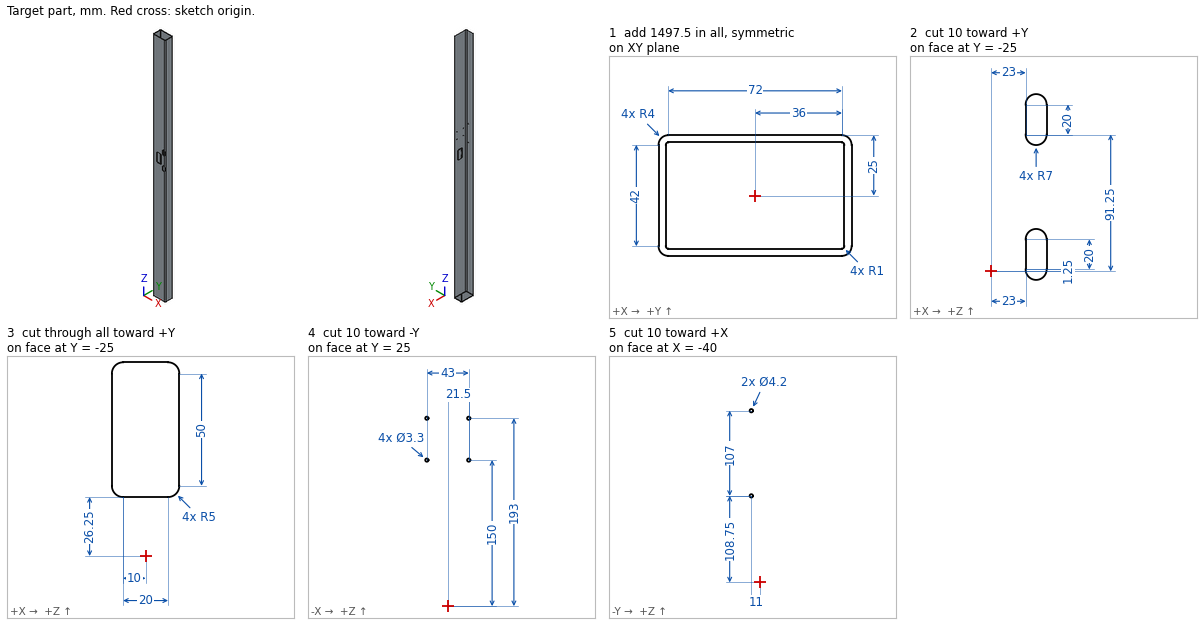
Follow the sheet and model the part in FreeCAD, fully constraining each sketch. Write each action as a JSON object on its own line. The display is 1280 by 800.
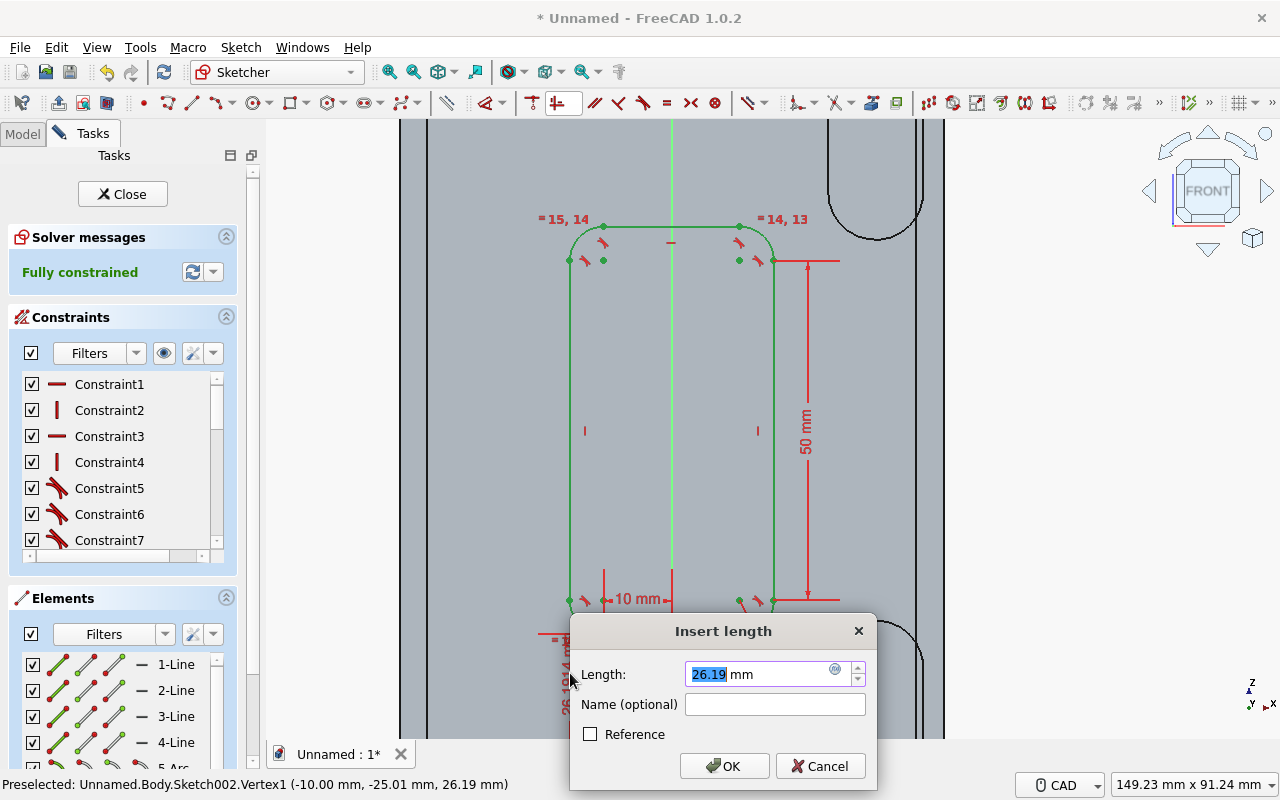
{"action": "type", "text": "26.25"}
{"action": "key", "text": "Return"}
{"action": "key", "text": "Escape"}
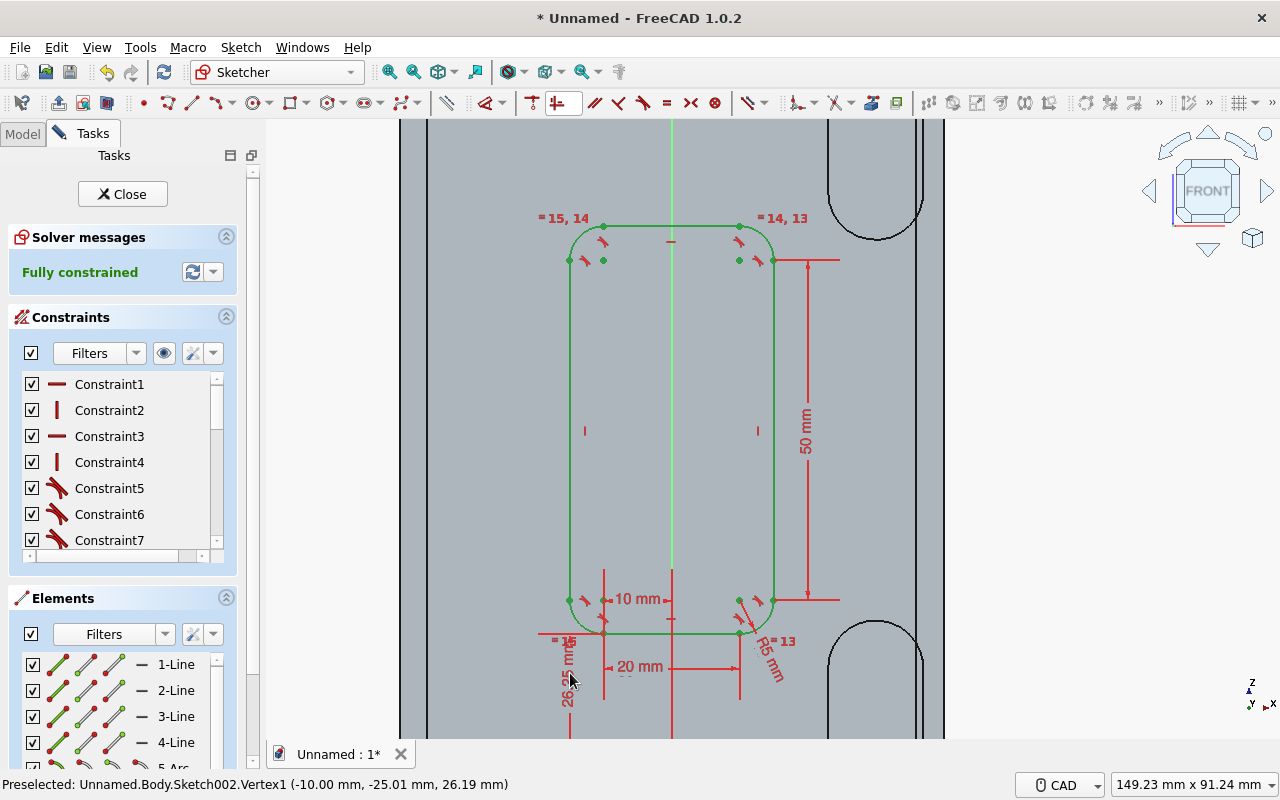
{"action": "left_click", "coordinate": [123, 194]}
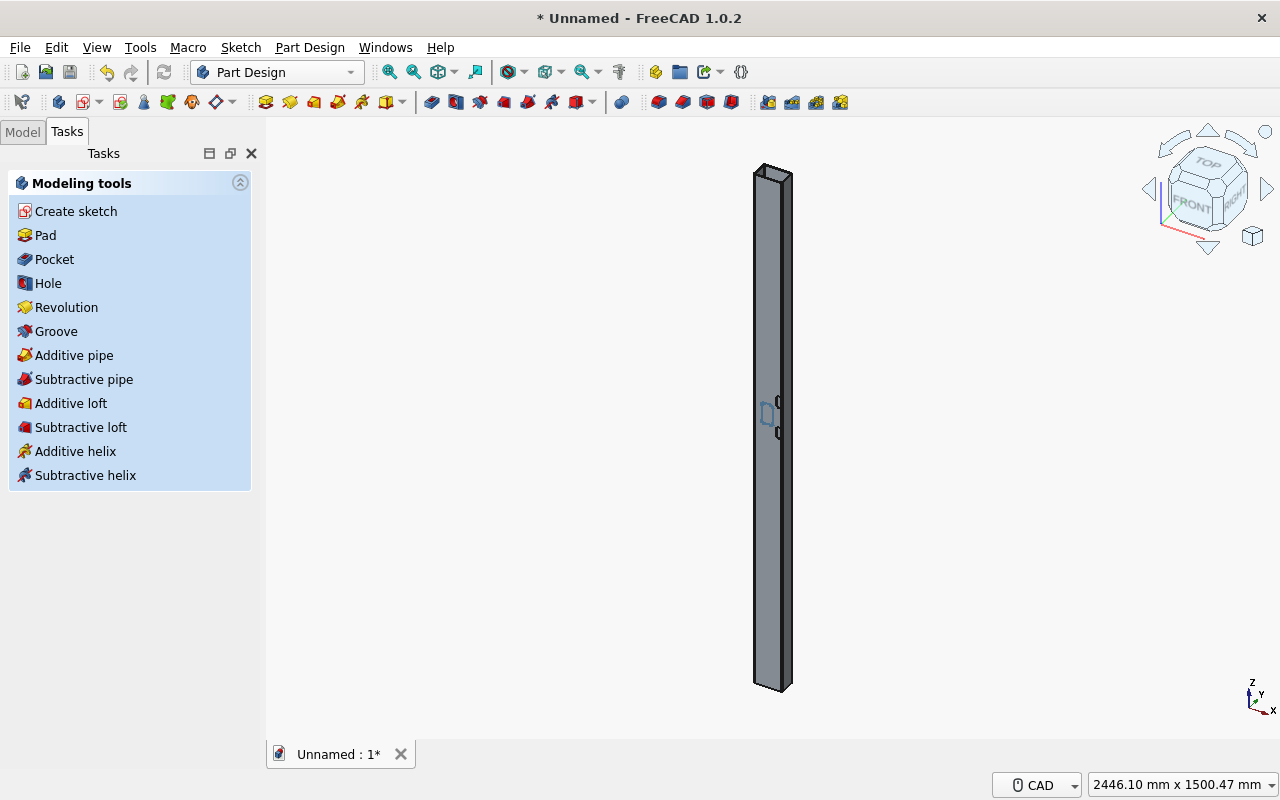
{"action": "left_click", "coordinate": [432, 102]}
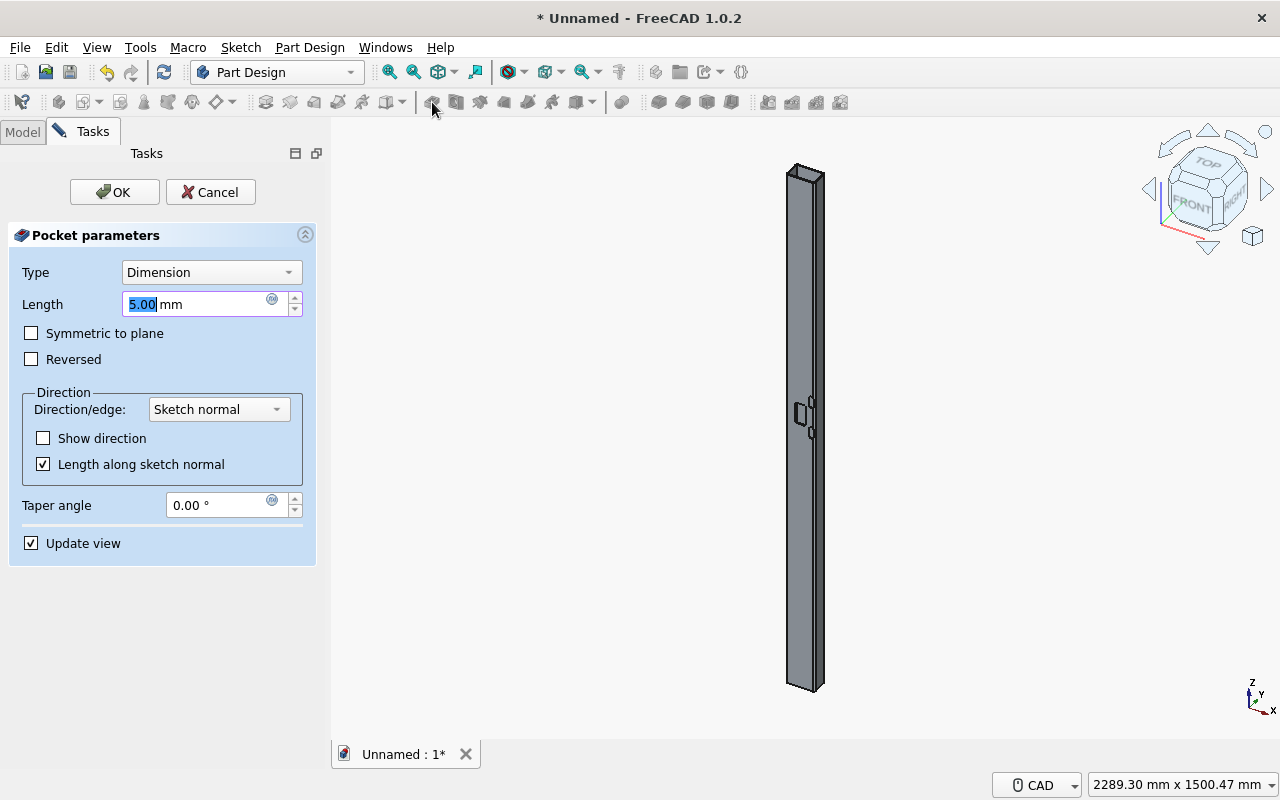
{"action": "left_click", "coordinate": [212, 272]}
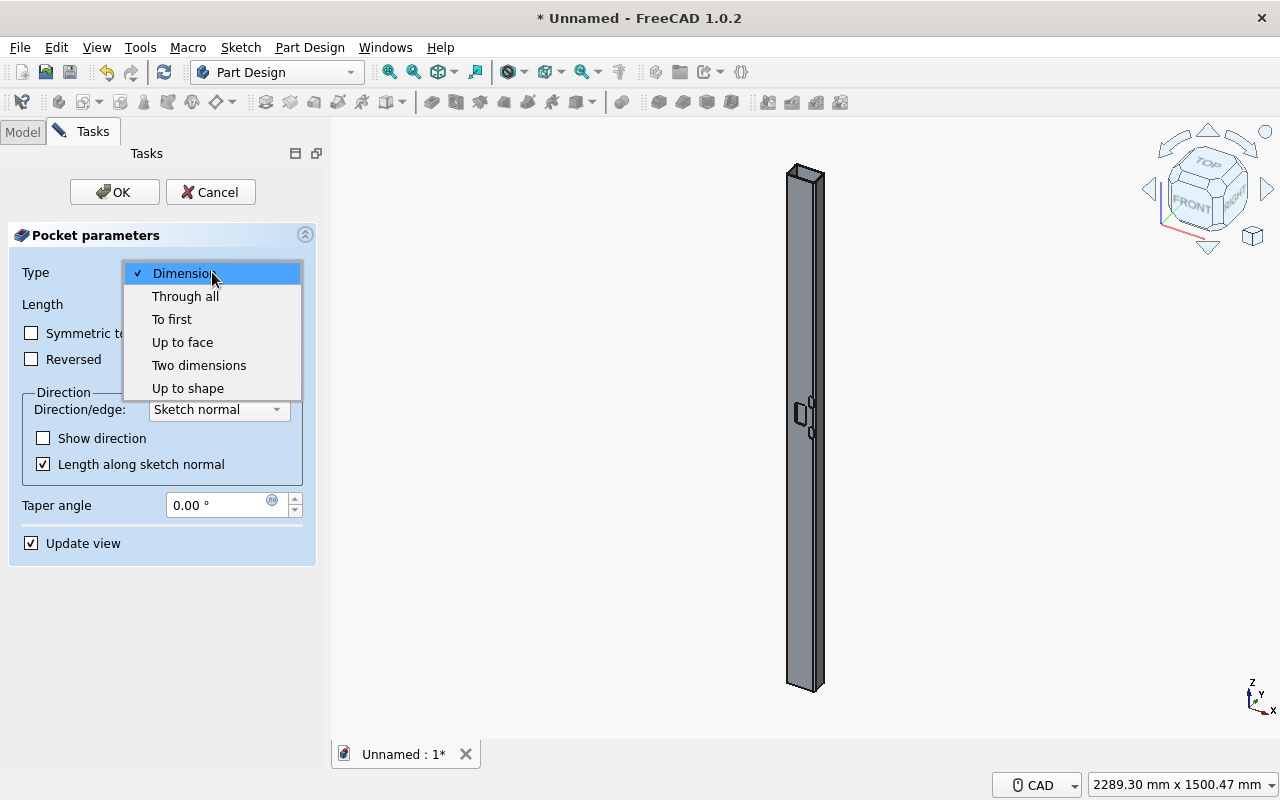
{"action": "left_click", "coordinate": [212, 296]}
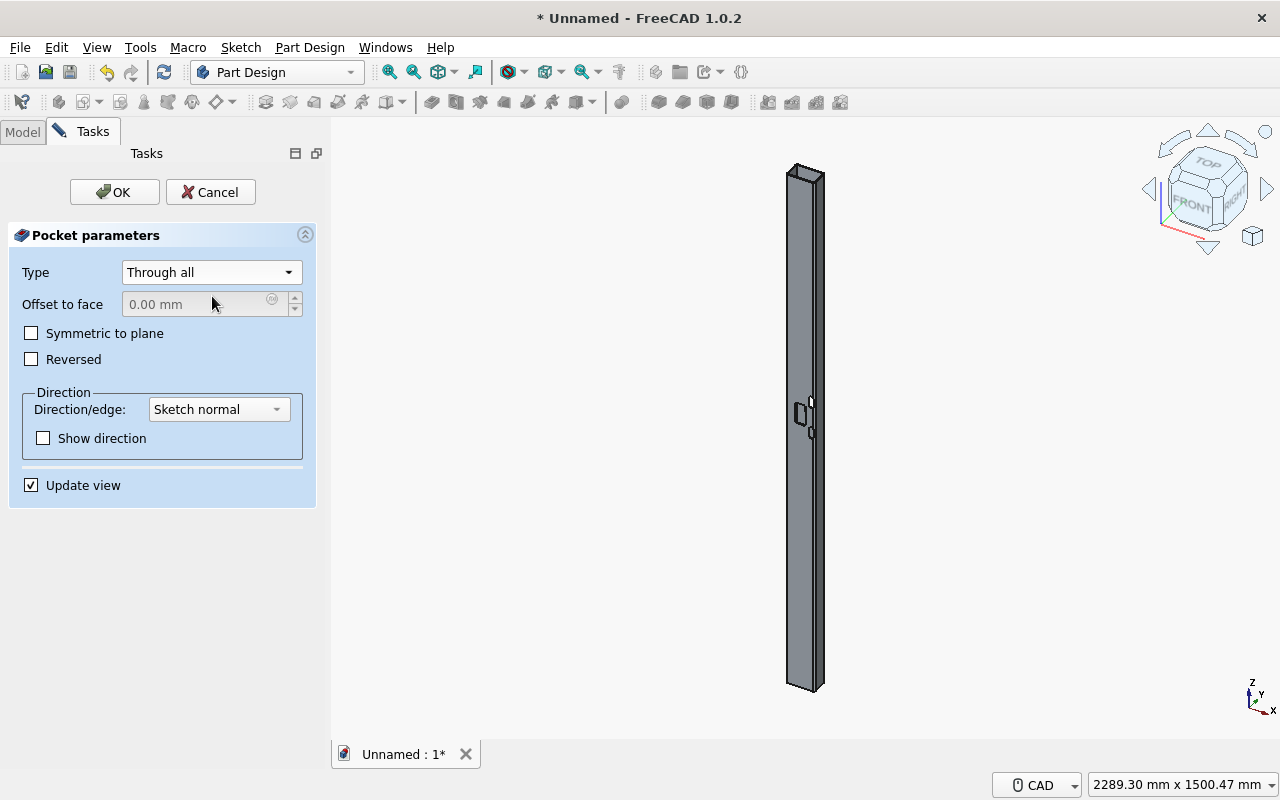
{"action": "left_click", "coordinate": [115, 192]}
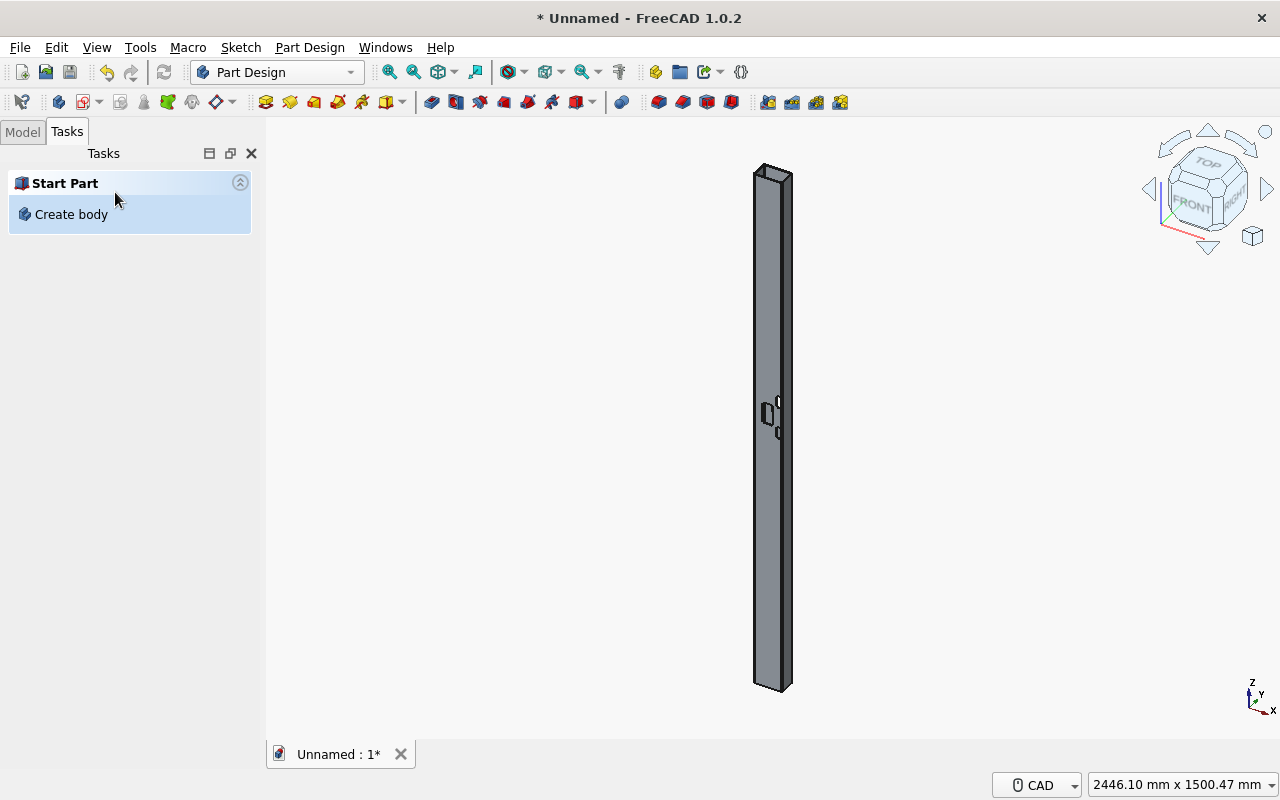
{"action": "key", "text": "4"}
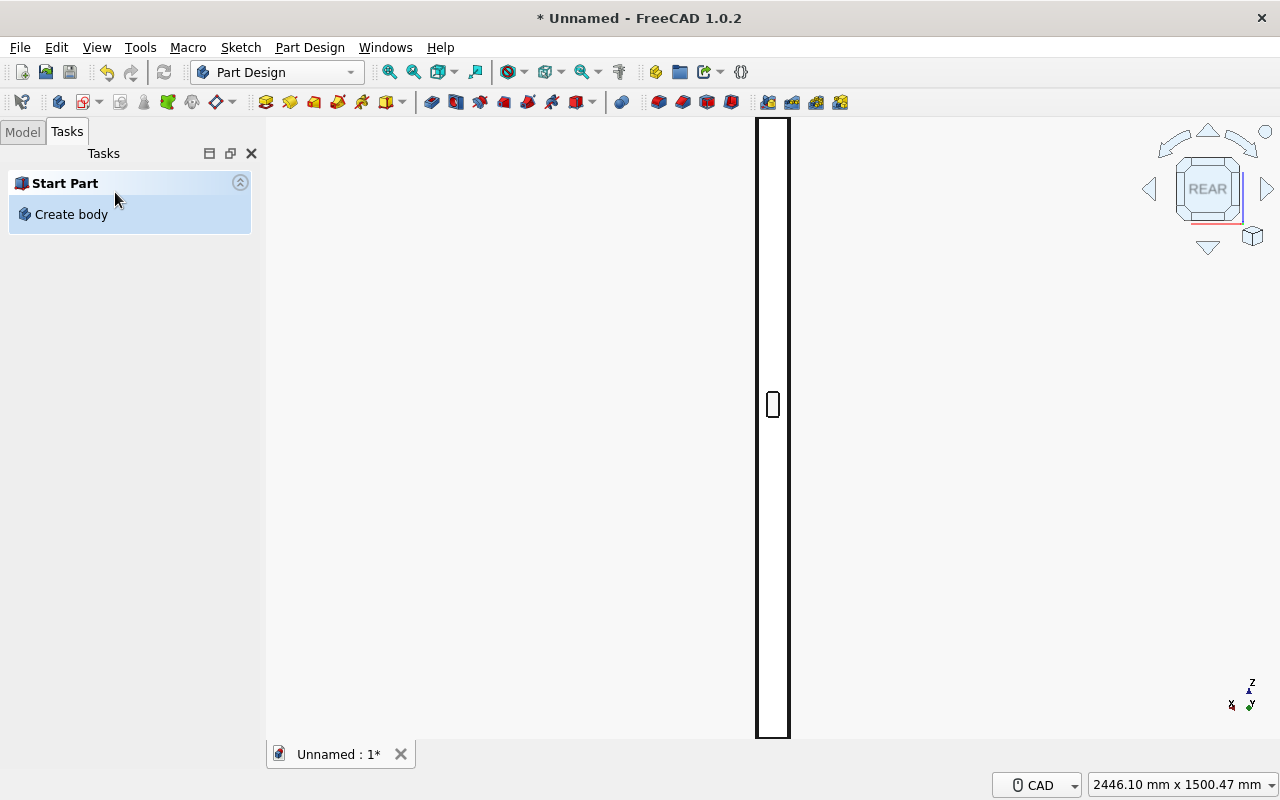
{"action": "left_click", "coordinate": [773, 161]}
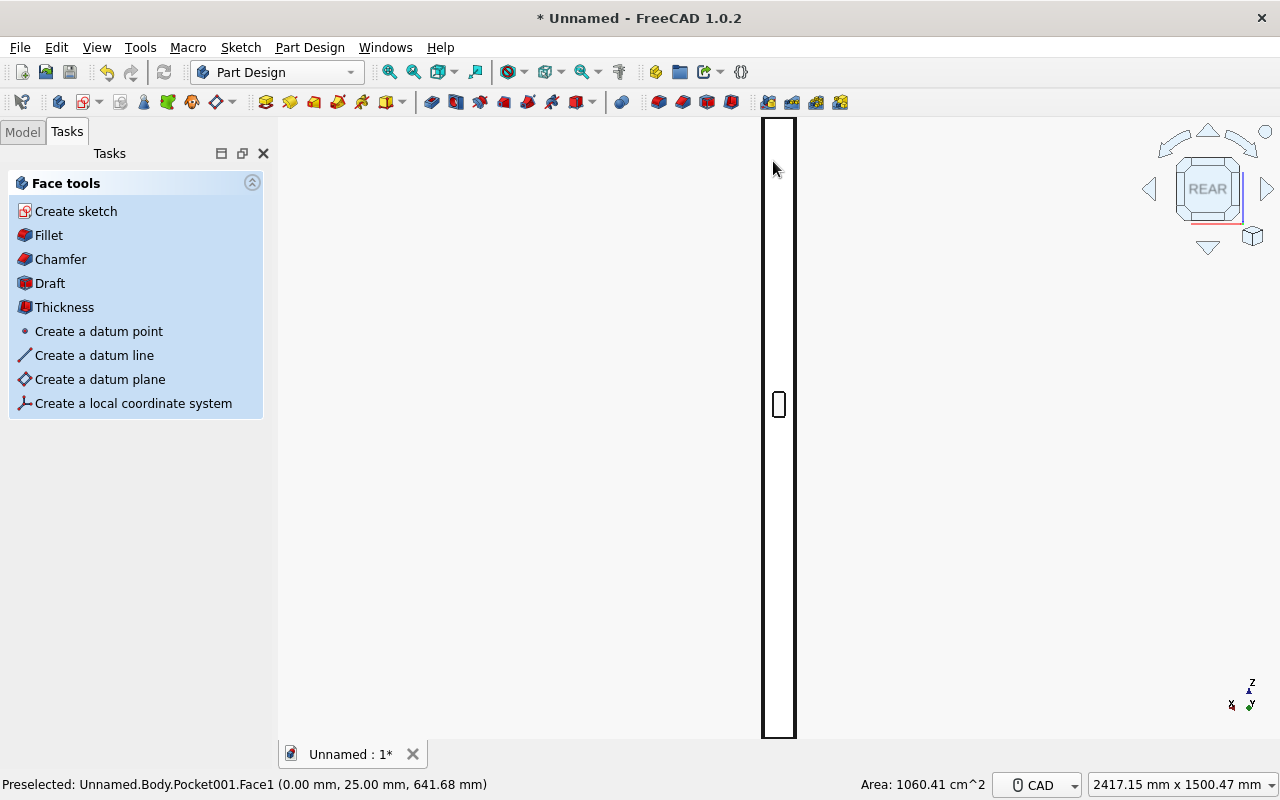
{"action": "left_click", "coordinate": [84, 102]}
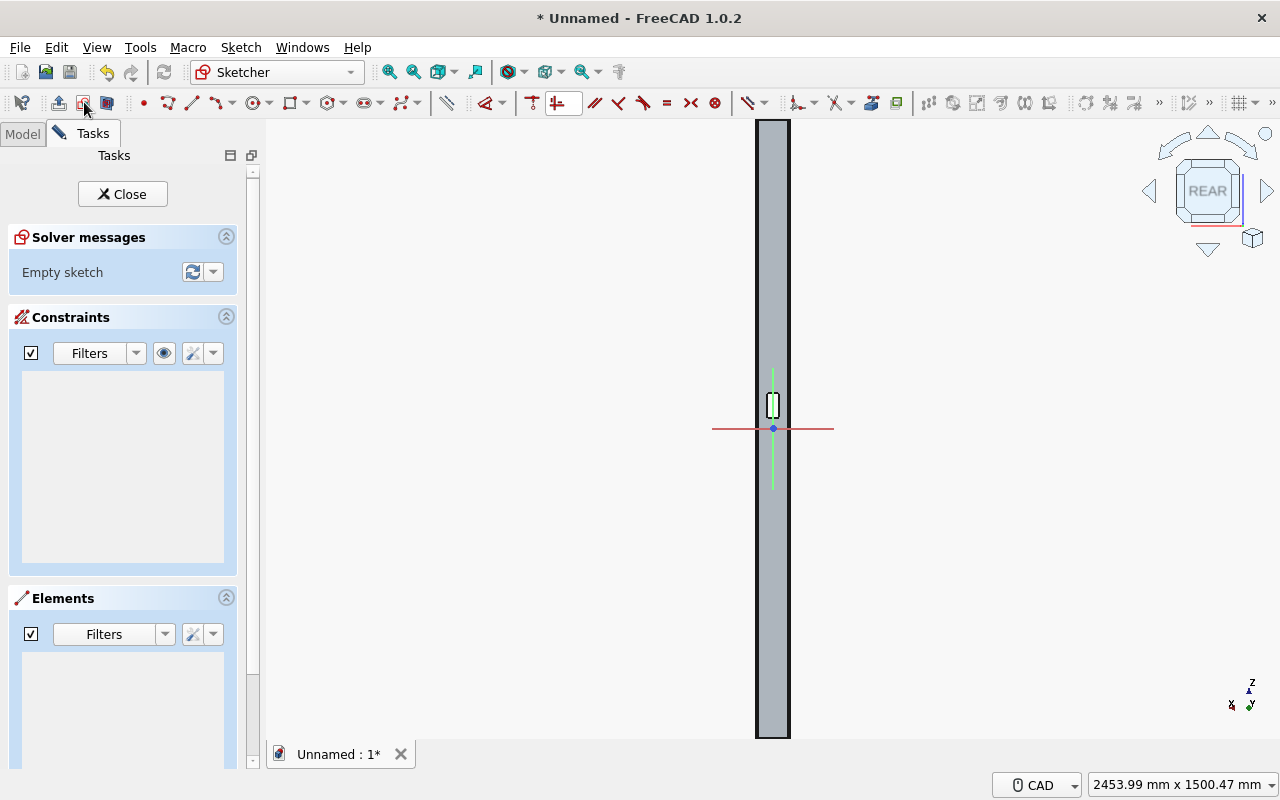
{"action": "scroll", "coordinate": [777, 354], "scroll_direction": "up", "scroll_amount": 15}